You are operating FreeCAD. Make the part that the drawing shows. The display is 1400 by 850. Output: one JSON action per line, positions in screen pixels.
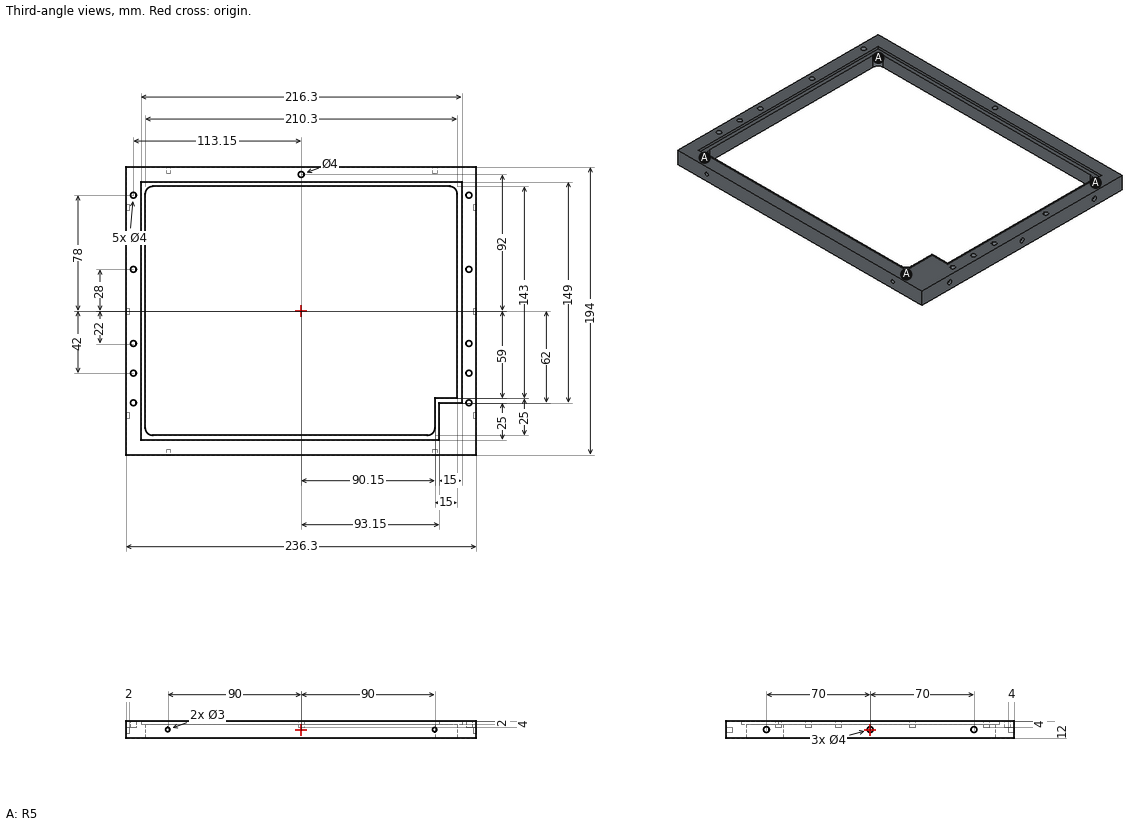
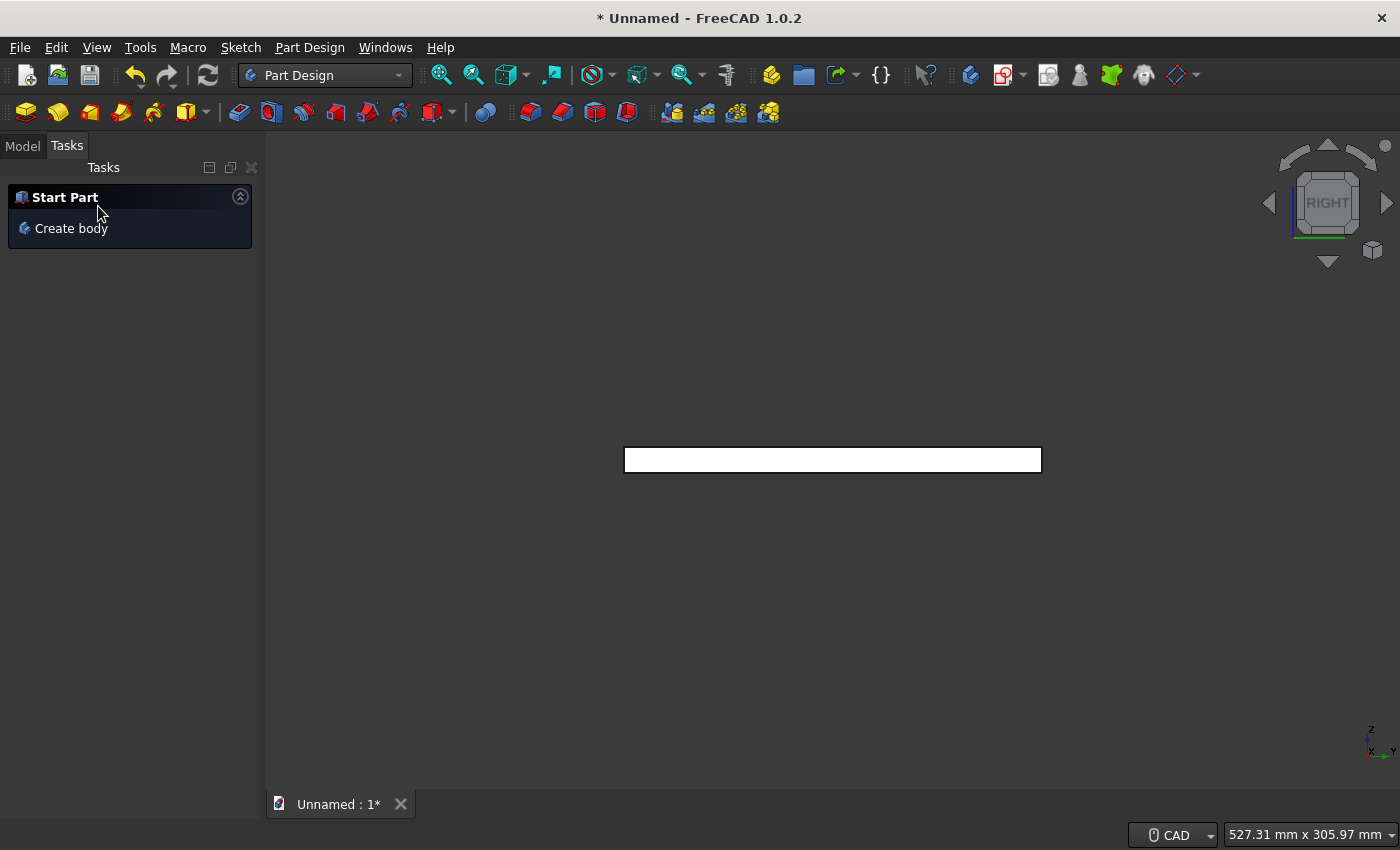
{"action": "left_click", "coordinate": [442, 76]}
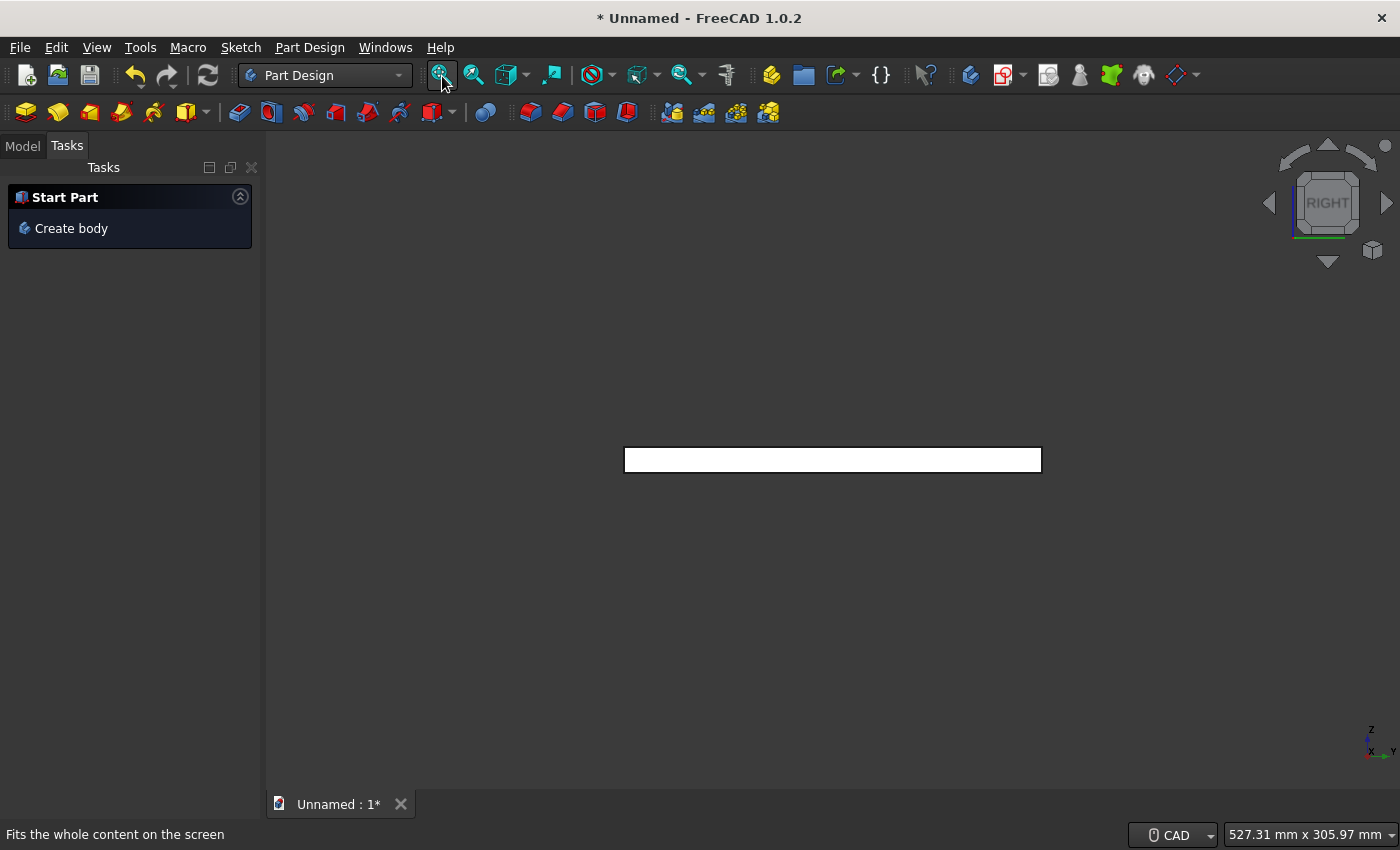
{"action": "key", "text": "6"}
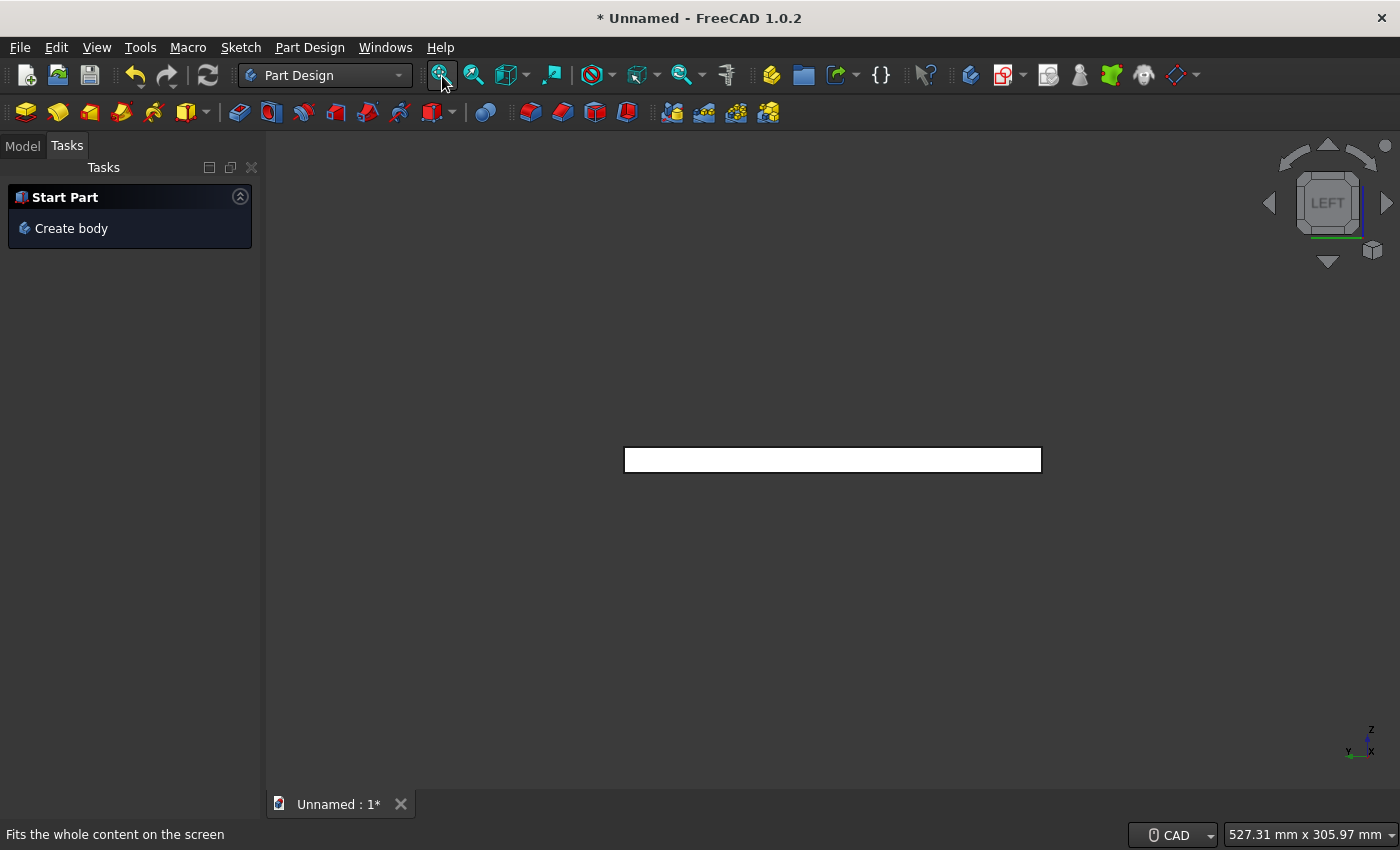
{"action": "left_click", "coordinate": [442, 76]}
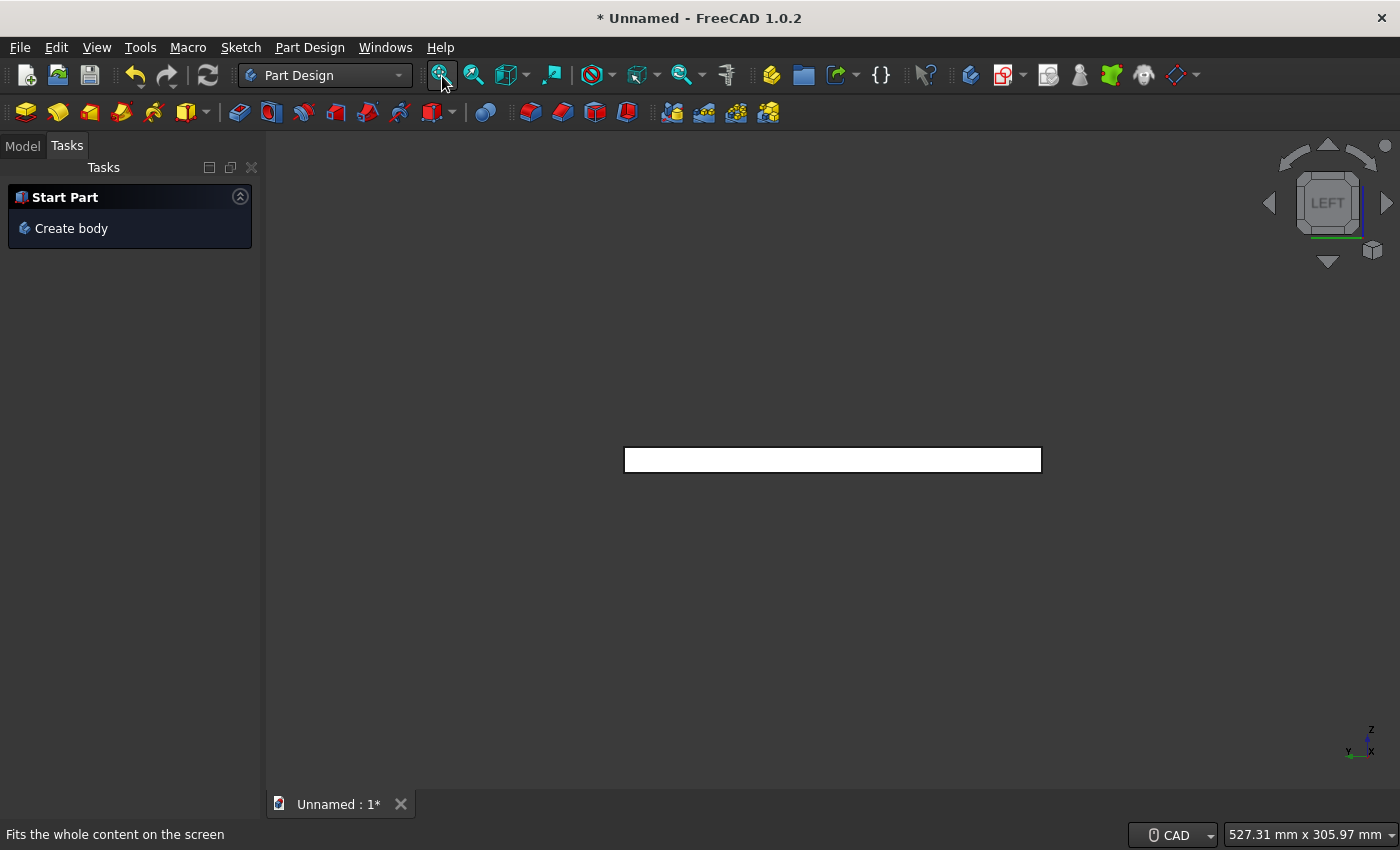
{"action": "left_click", "coordinate": [654, 459]}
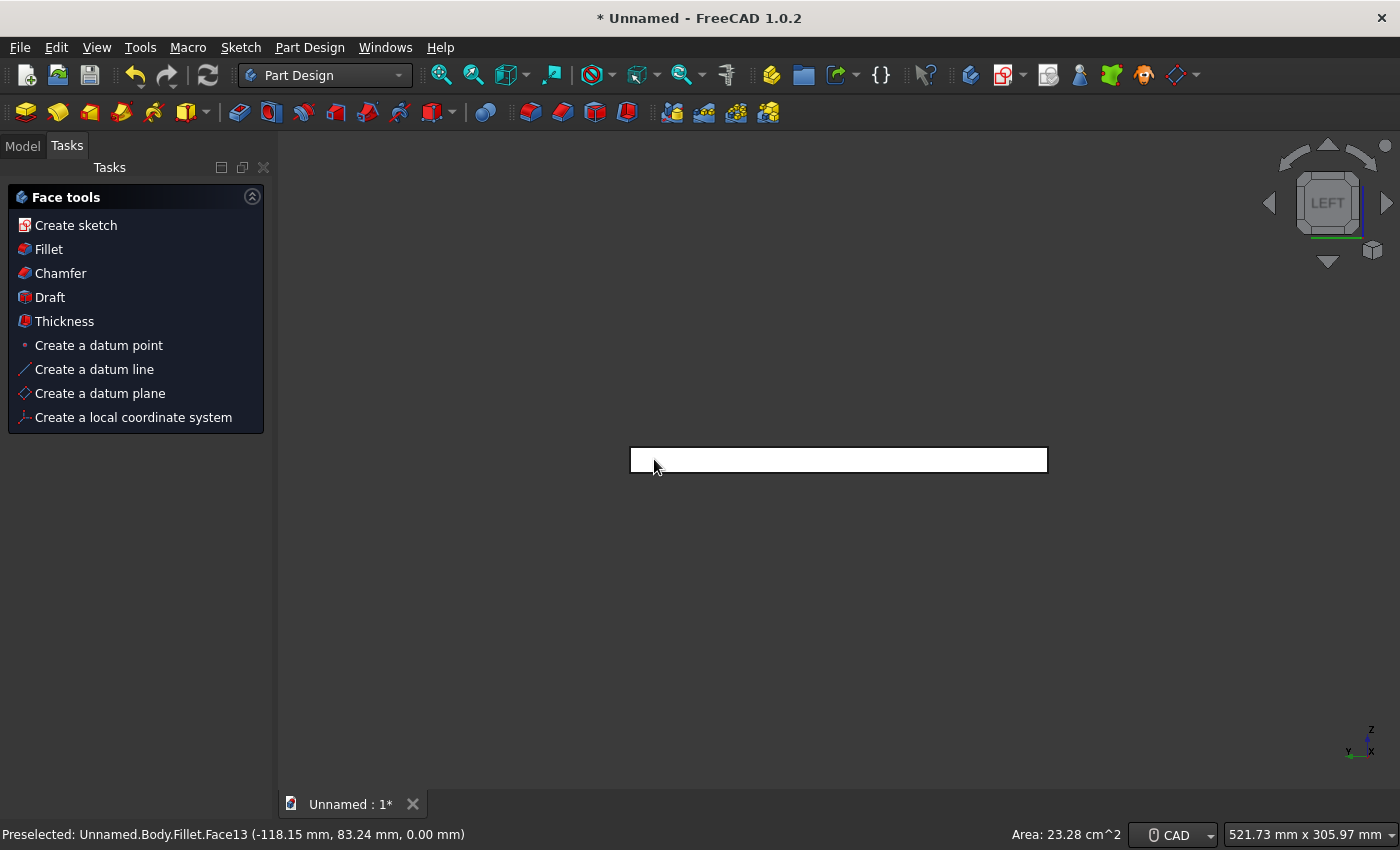
{"action": "left_click", "coordinate": [1004, 76]}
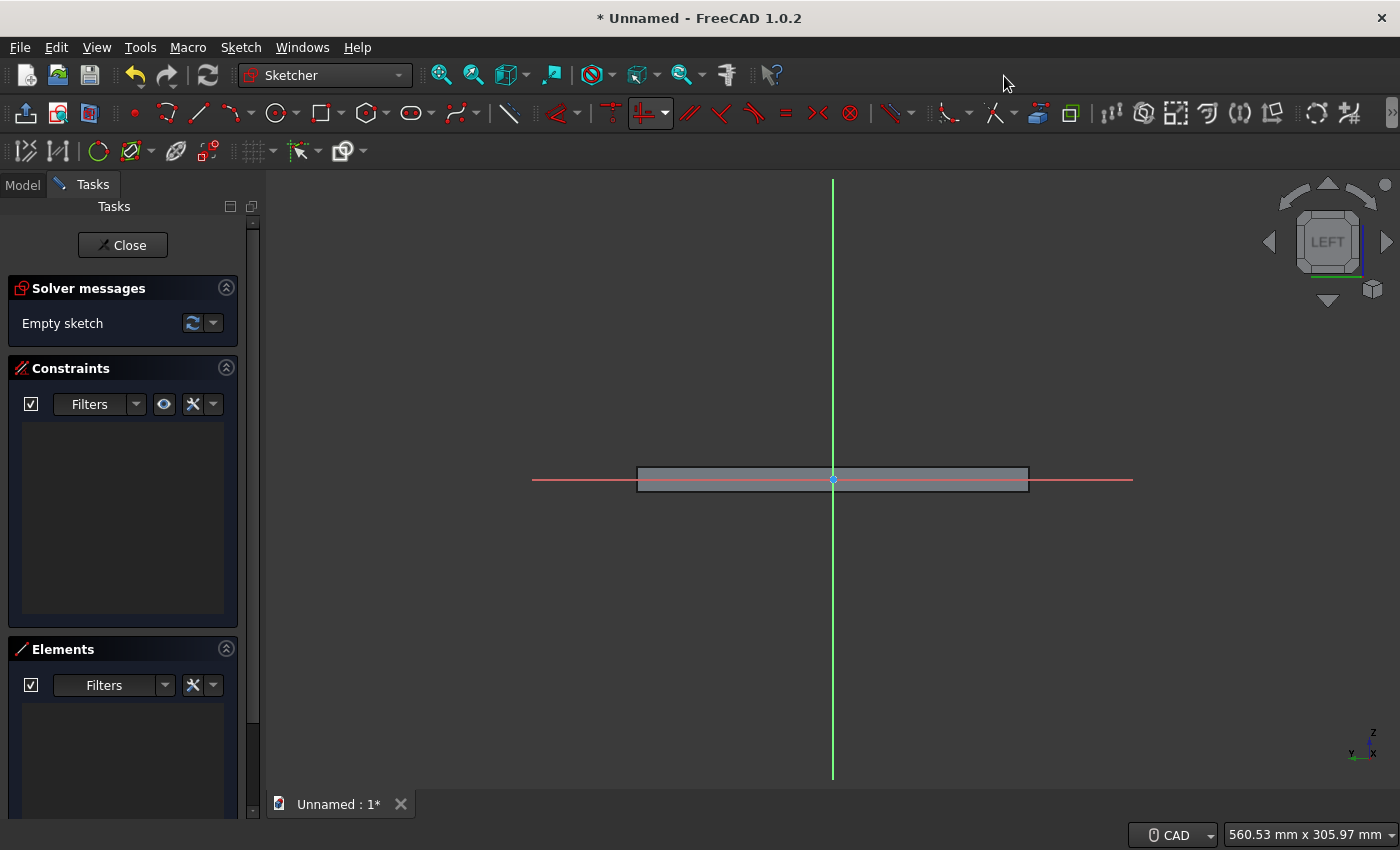
{"action": "scroll", "coordinate": [889, 480], "scroll_direction": "up", "scroll_amount": 4}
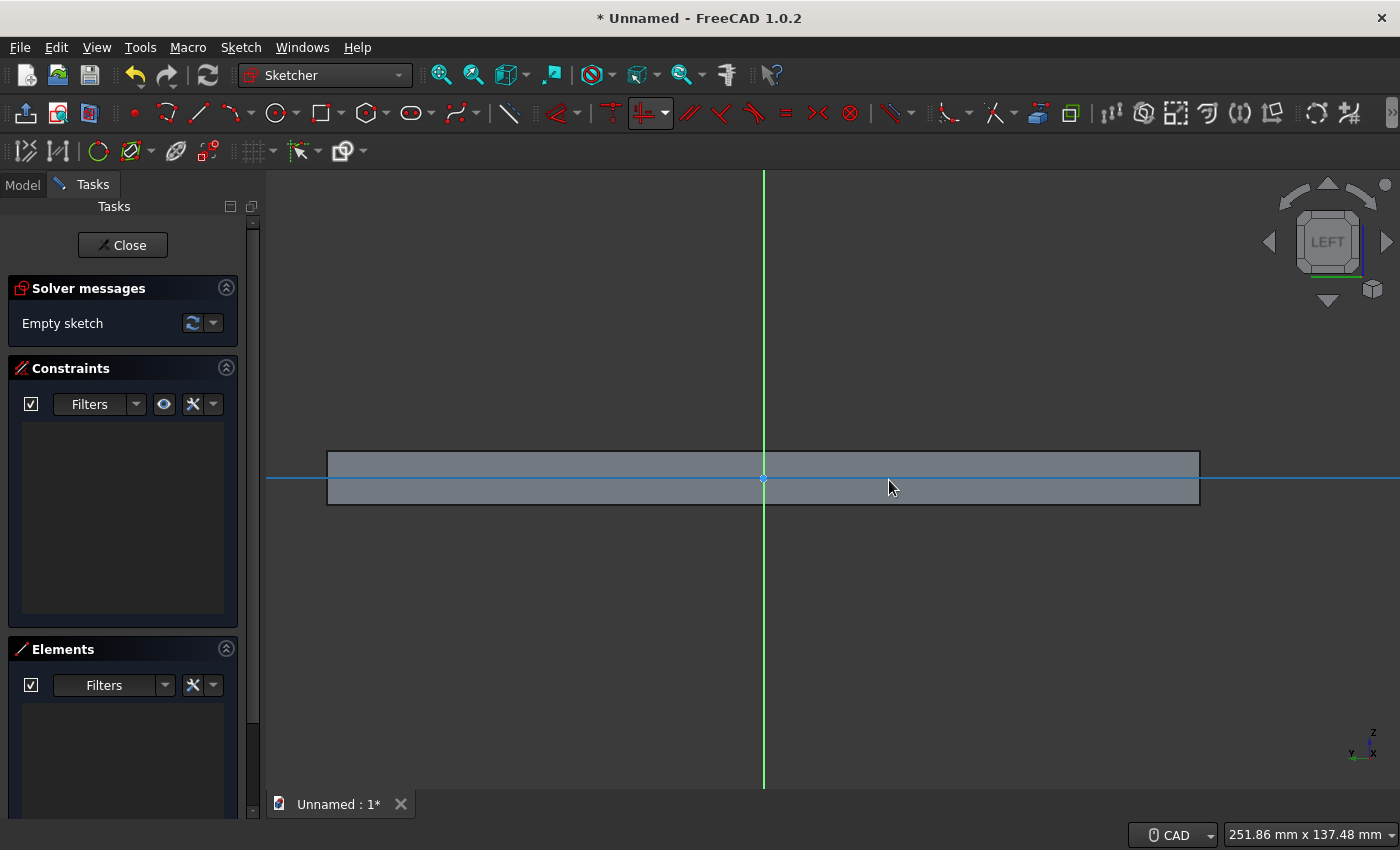
{"action": "left_click", "coordinate": [276, 114]}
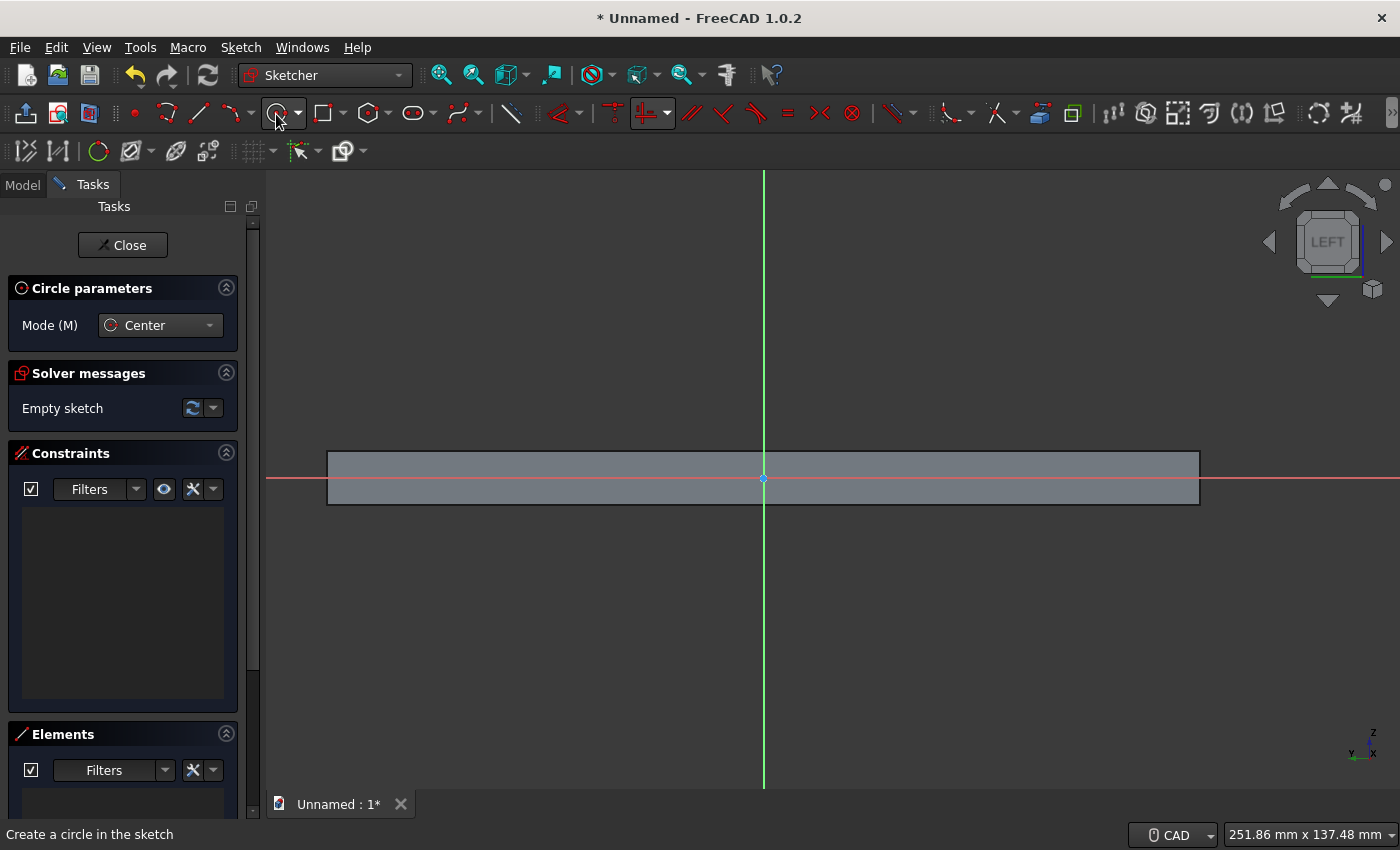
{"action": "scroll", "coordinate": [764, 478], "scroll_direction": "up", "scroll_amount": 5}